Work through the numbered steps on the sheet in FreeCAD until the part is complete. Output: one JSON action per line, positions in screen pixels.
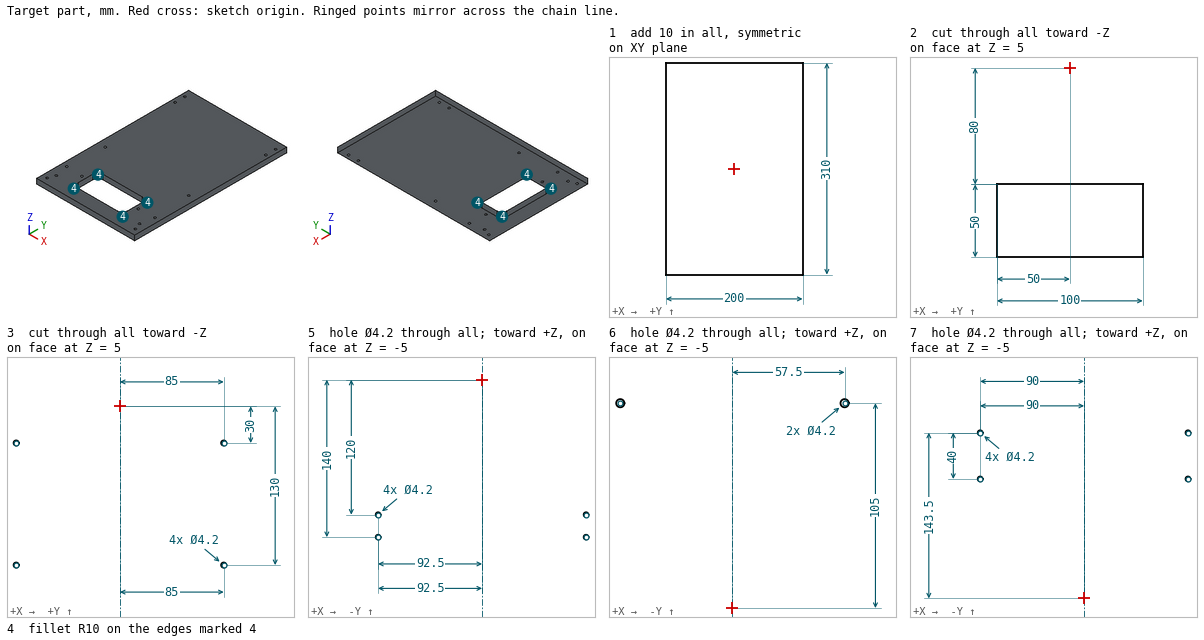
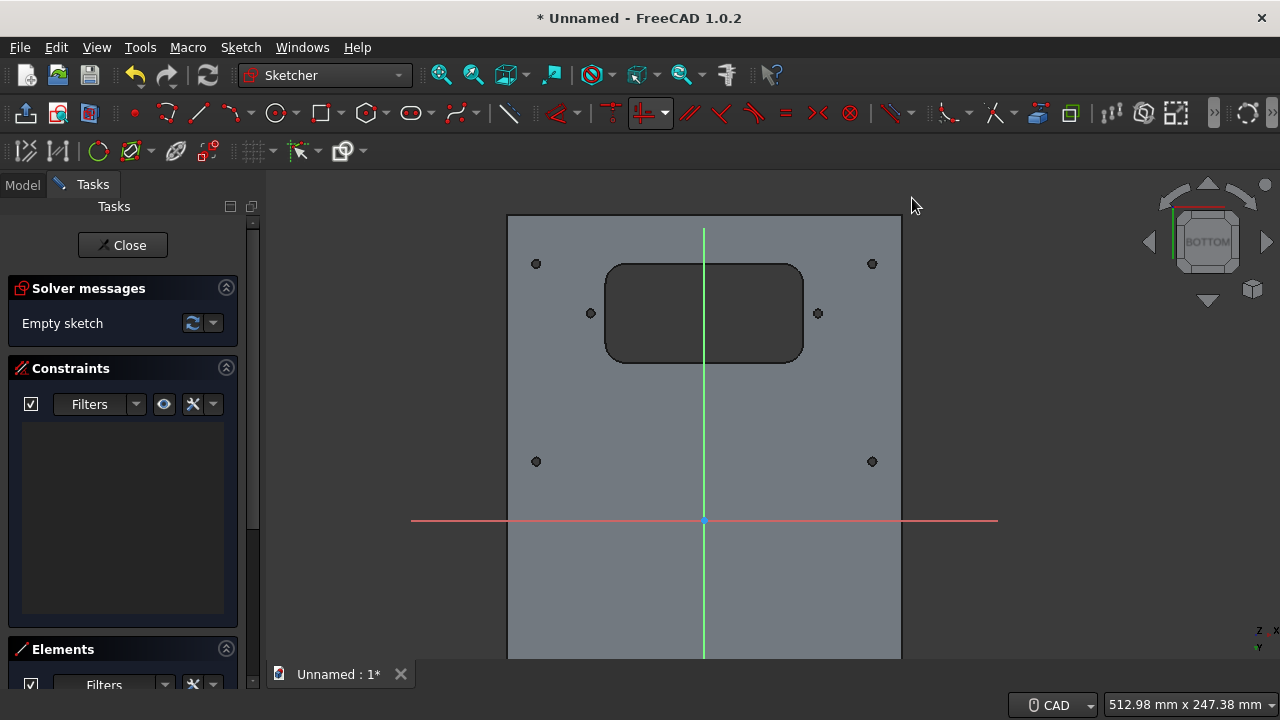
{"action": "left_click", "coordinate": [276, 114]}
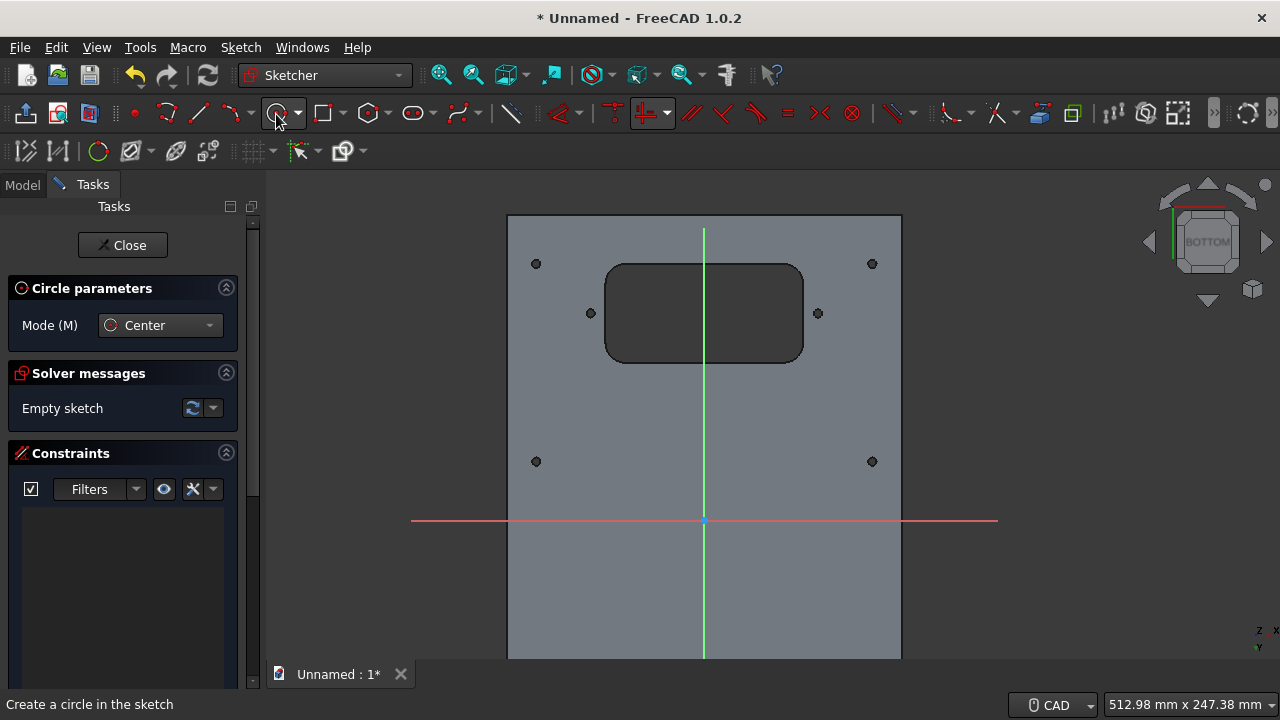
{"action": "scroll", "coordinate": [526, 237], "scroll_direction": "up", "scroll_amount": 9}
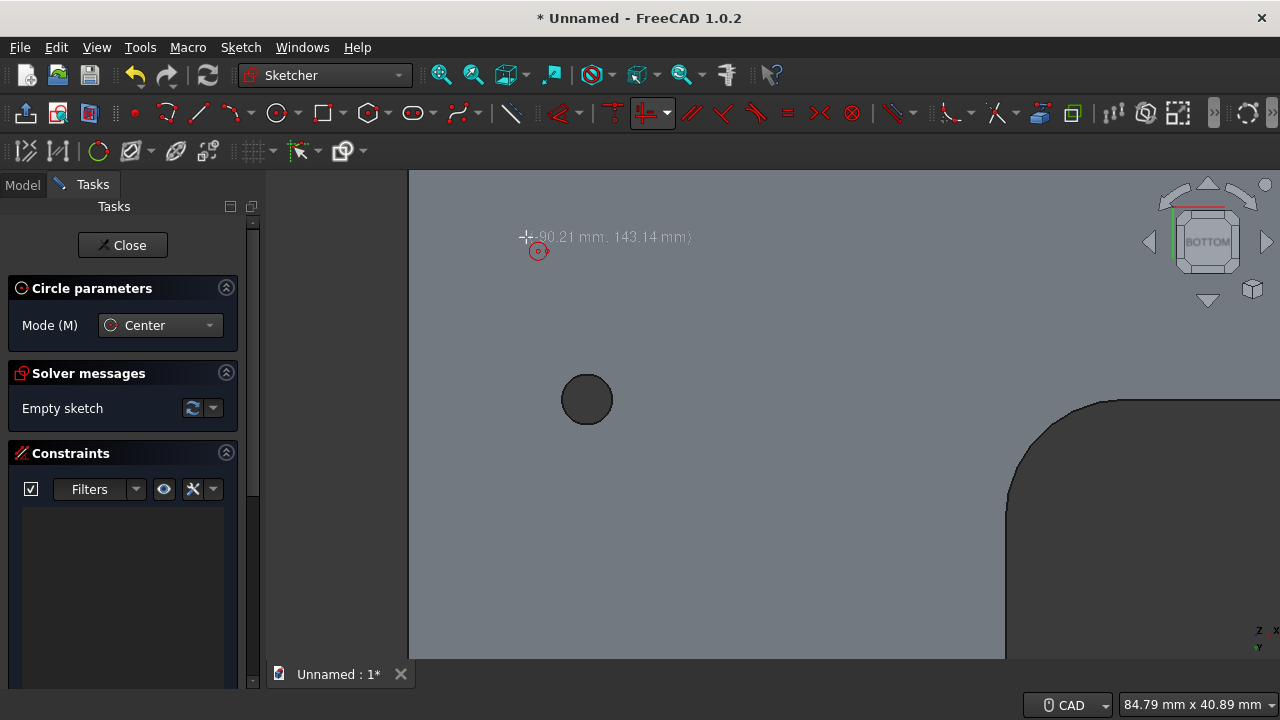
{"action": "scroll", "coordinate": [526, 282], "scroll_direction": "down", "scroll_amount": 9}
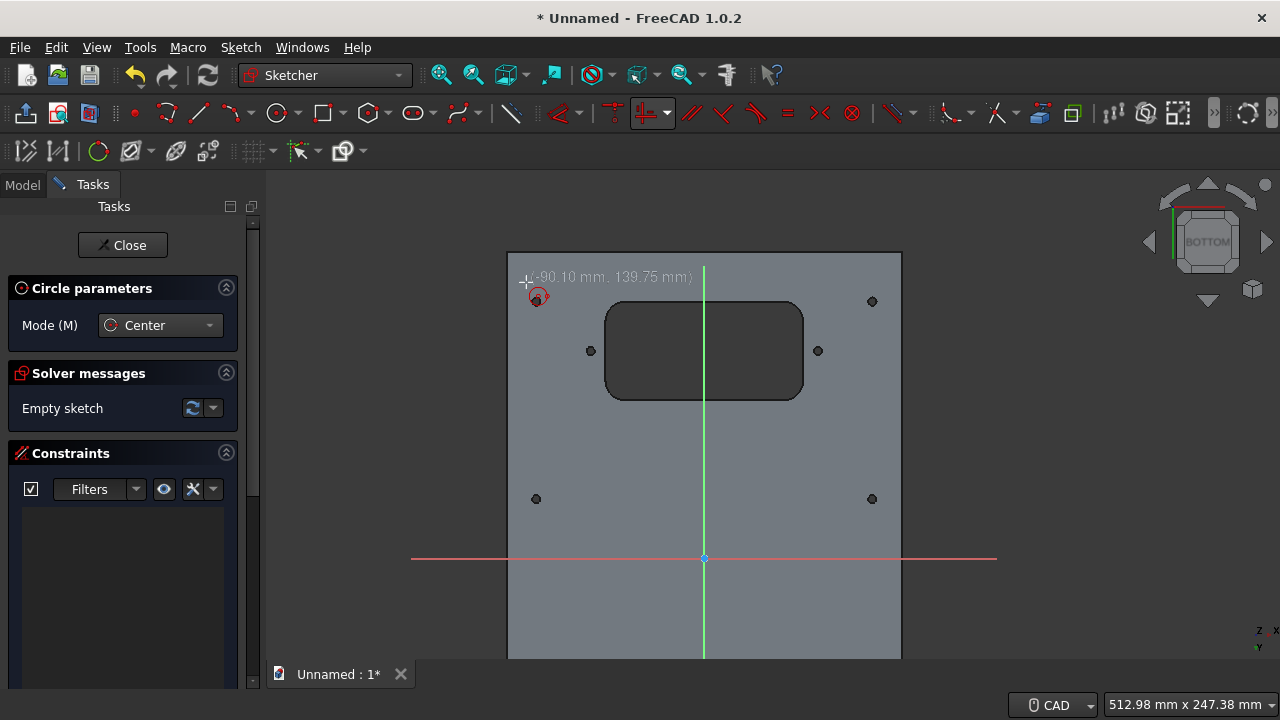
{"action": "left_click", "coordinate": [526, 275]}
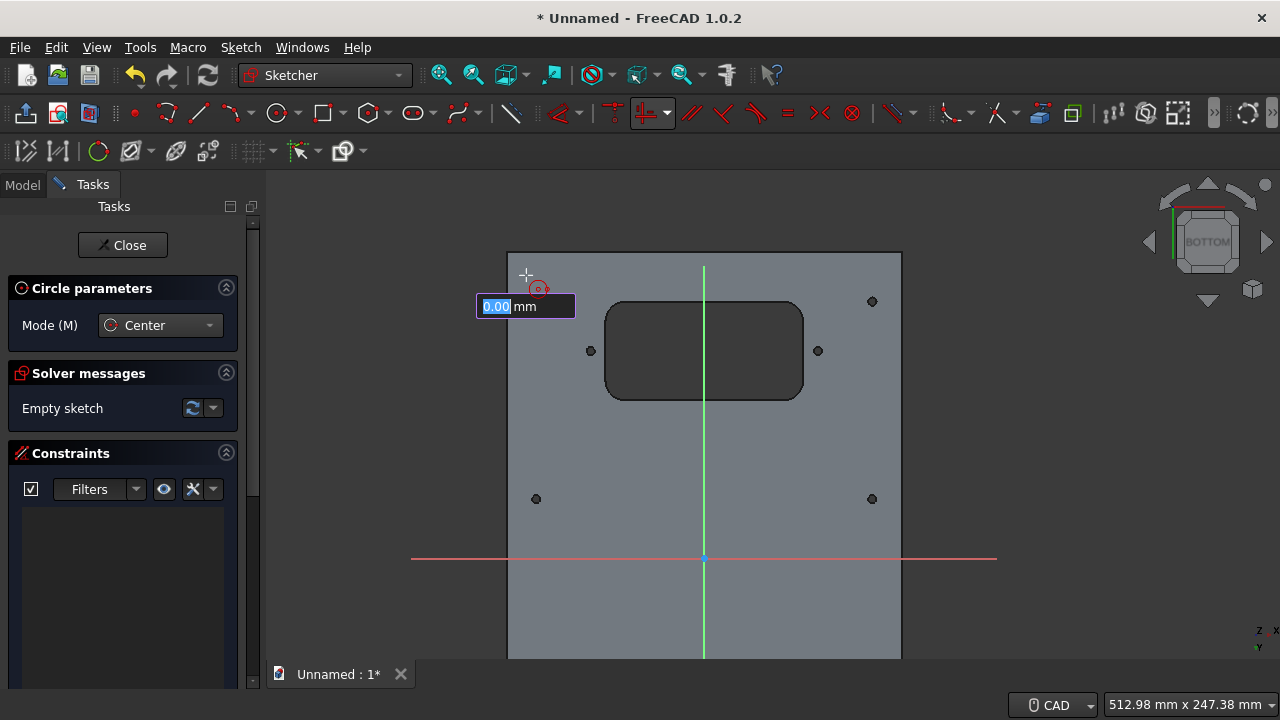
{"action": "scroll", "coordinate": [529, 272], "scroll_direction": "up", "scroll_amount": 7}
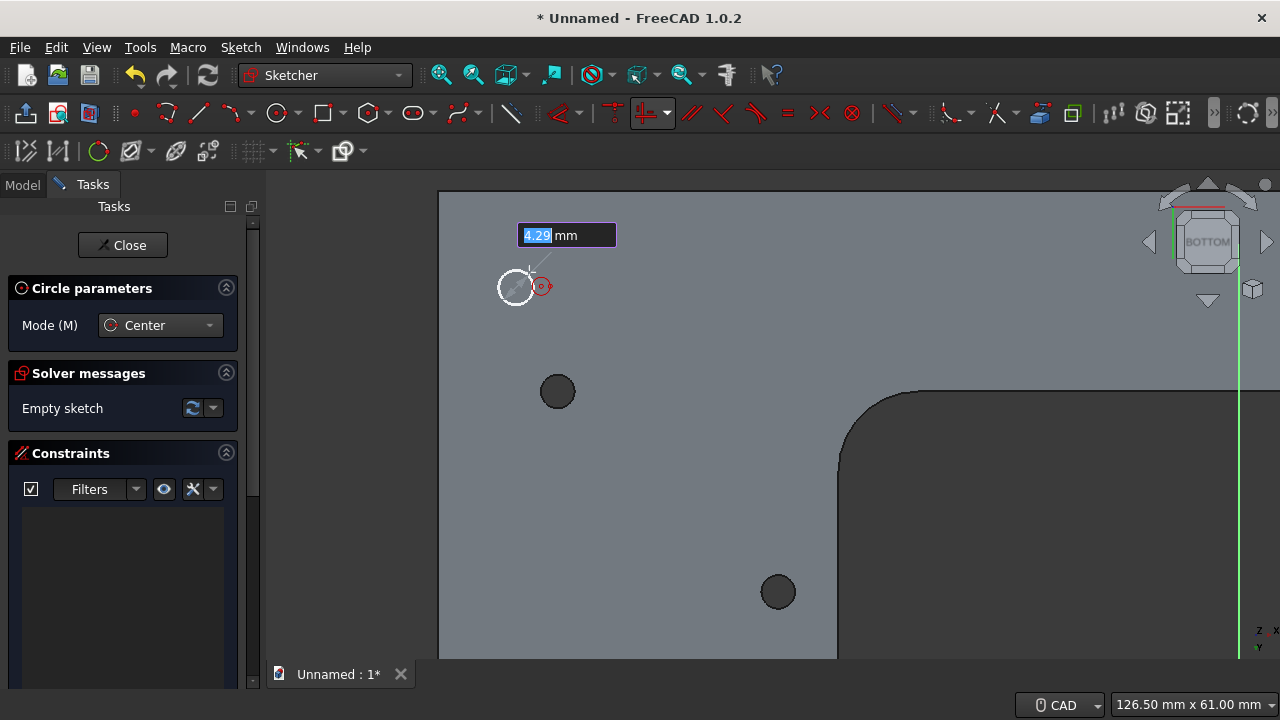
{"action": "left_click", "coordinate": [530, 271]}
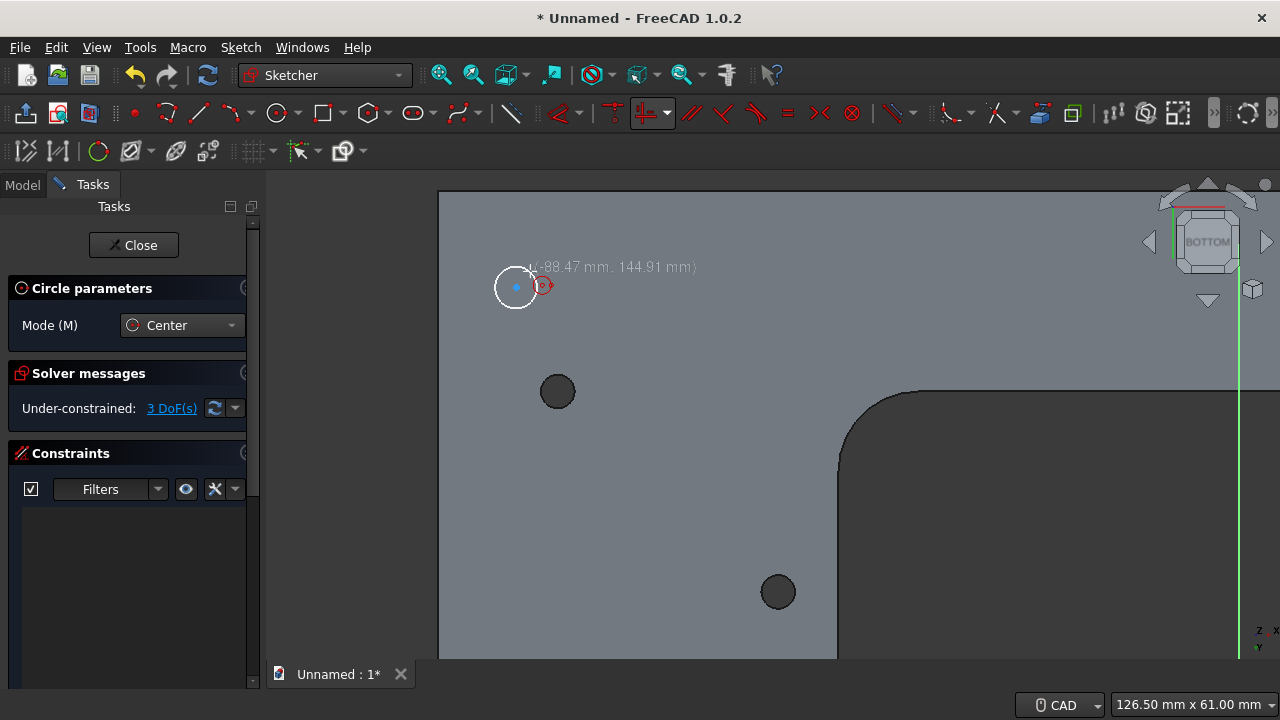
{"action": "scroll", "coordinate": [518, 604], "scroll_direction": "up", "scroll_amount": 2}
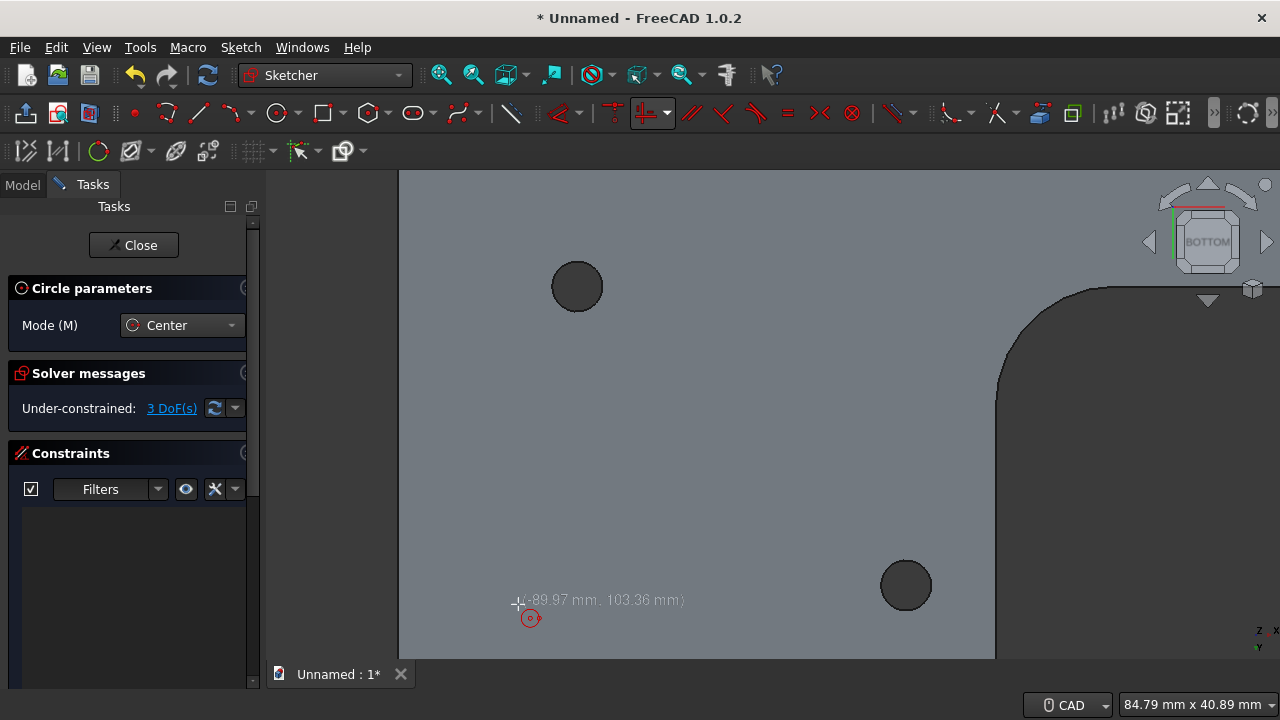
{"action": "scroll", "coordinate": [528, 304], "scroll_direction": "down", "scroll_amount": 9}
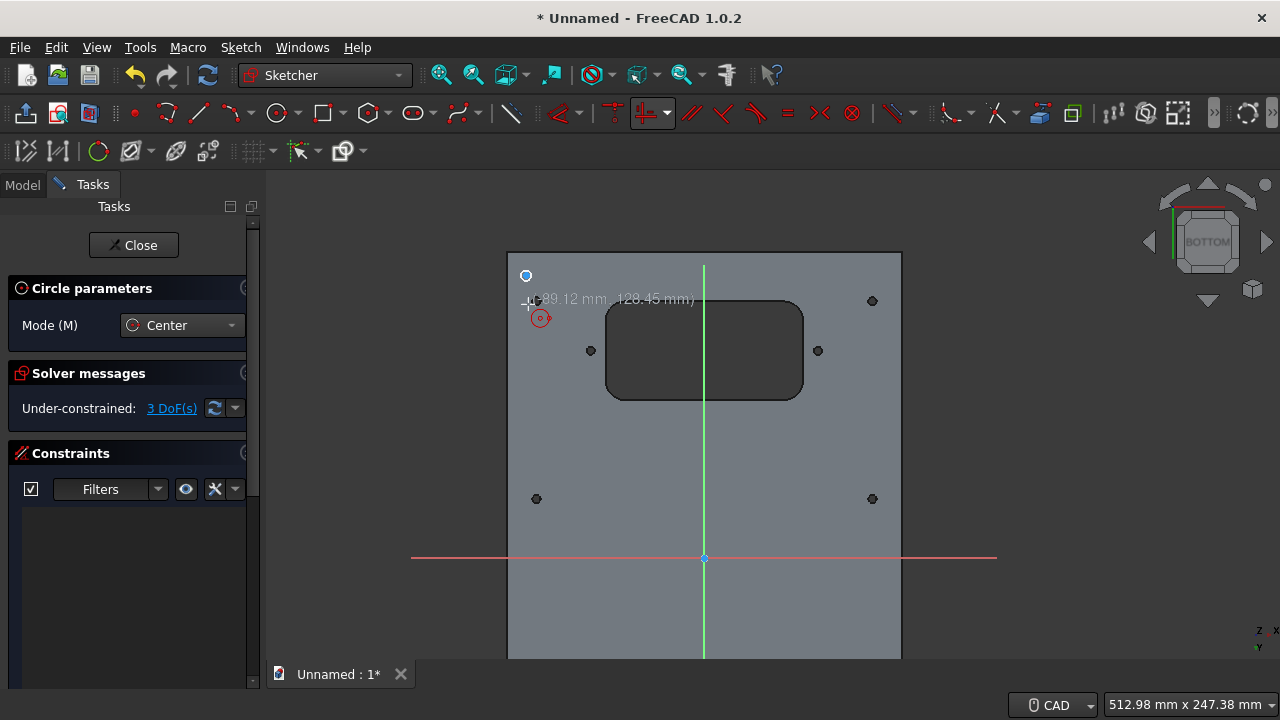
{"action": "left_click", "coordinate": [526, 354]}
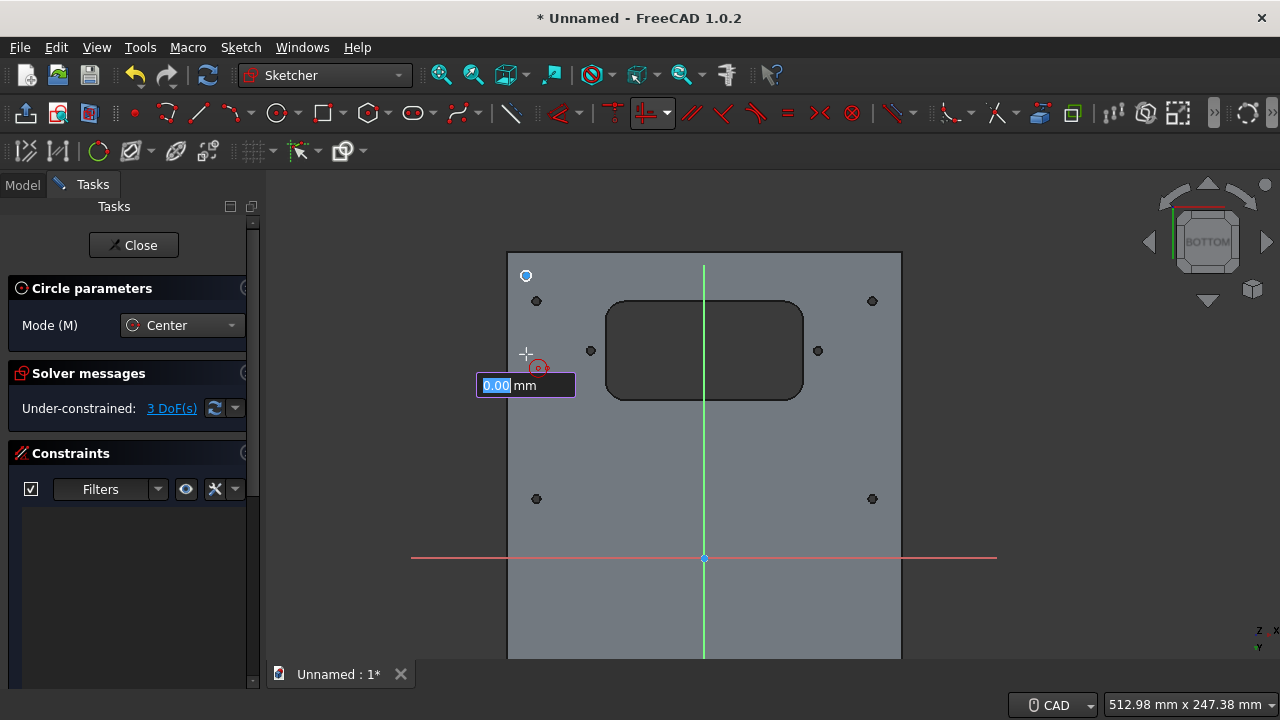
{"action": "scroll", "coordinate": [529, 351], "scroll_direction": "up", "scroll_amount": 7}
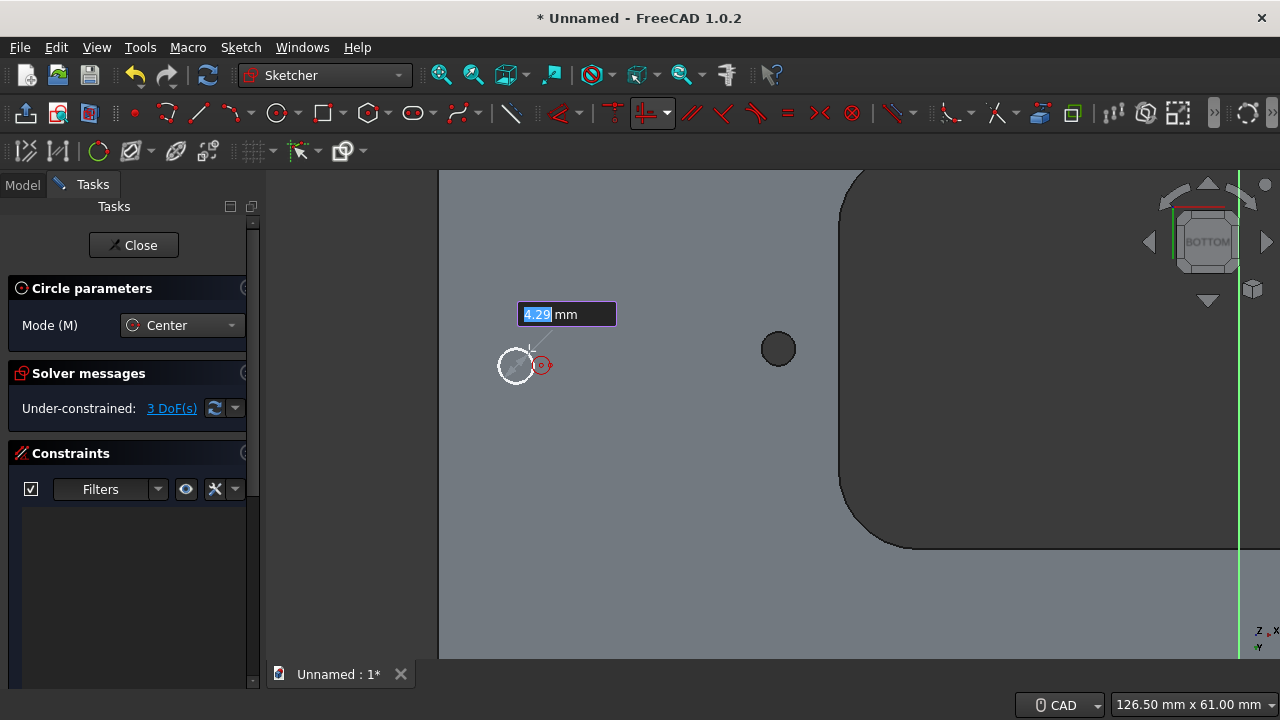
{"action": "left_click", "coordinate": [530, 349]}